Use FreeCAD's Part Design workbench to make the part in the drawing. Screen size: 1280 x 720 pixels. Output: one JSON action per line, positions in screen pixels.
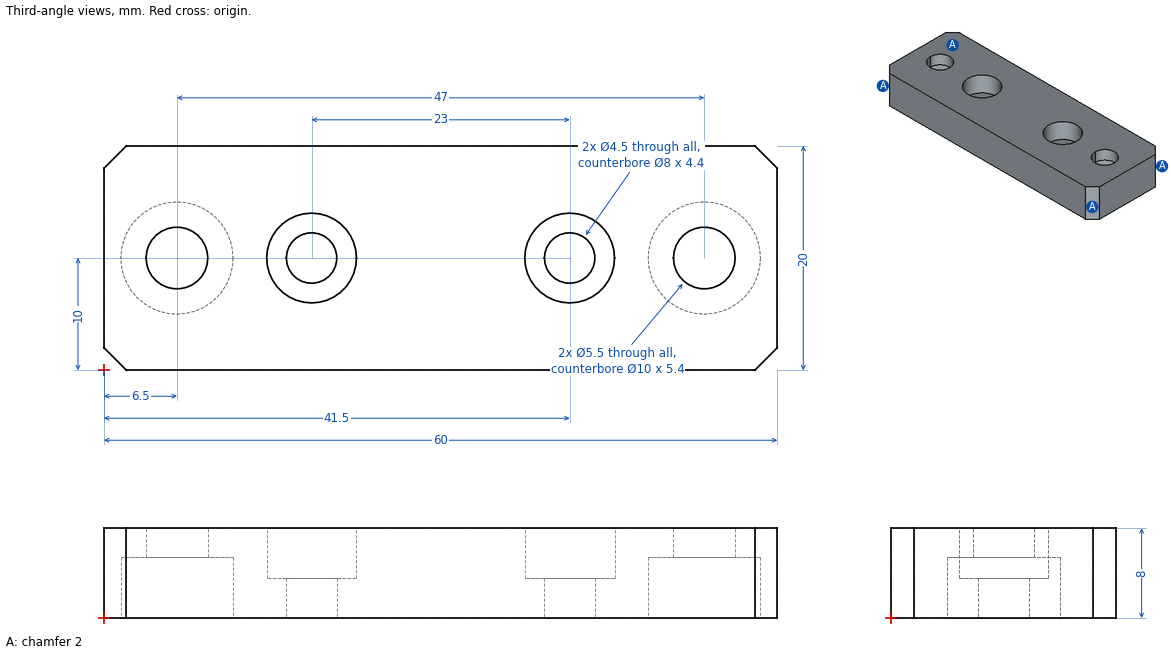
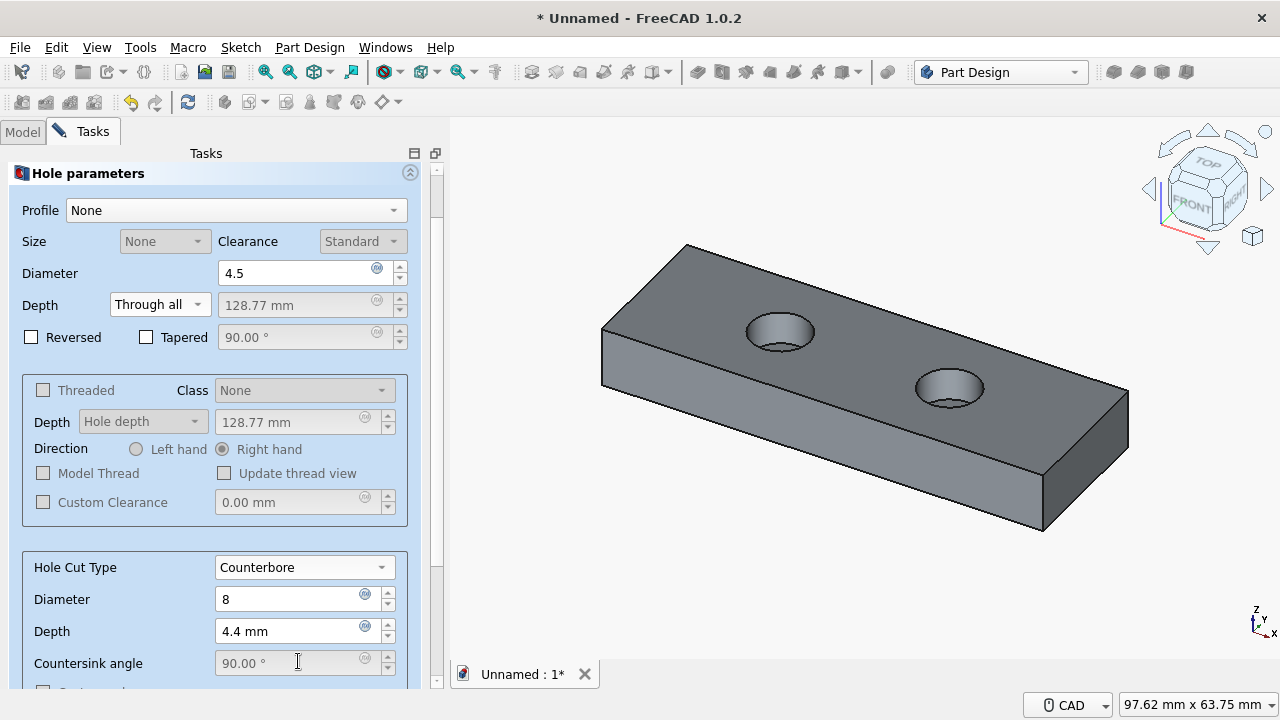
{"action": "scroll", "coordinate": [437, 426], "scroll_direction": "up", "scroll_amount": 2}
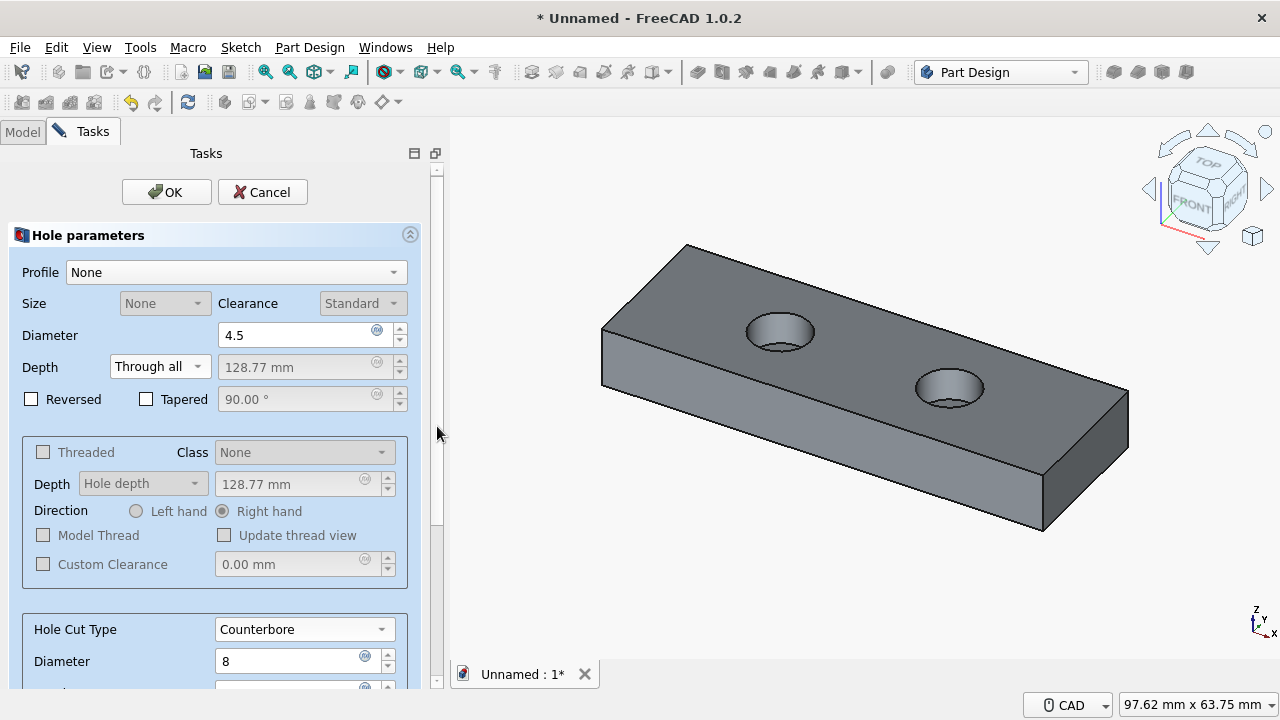
{"action": "left_click", "coordinate": [167, 192]}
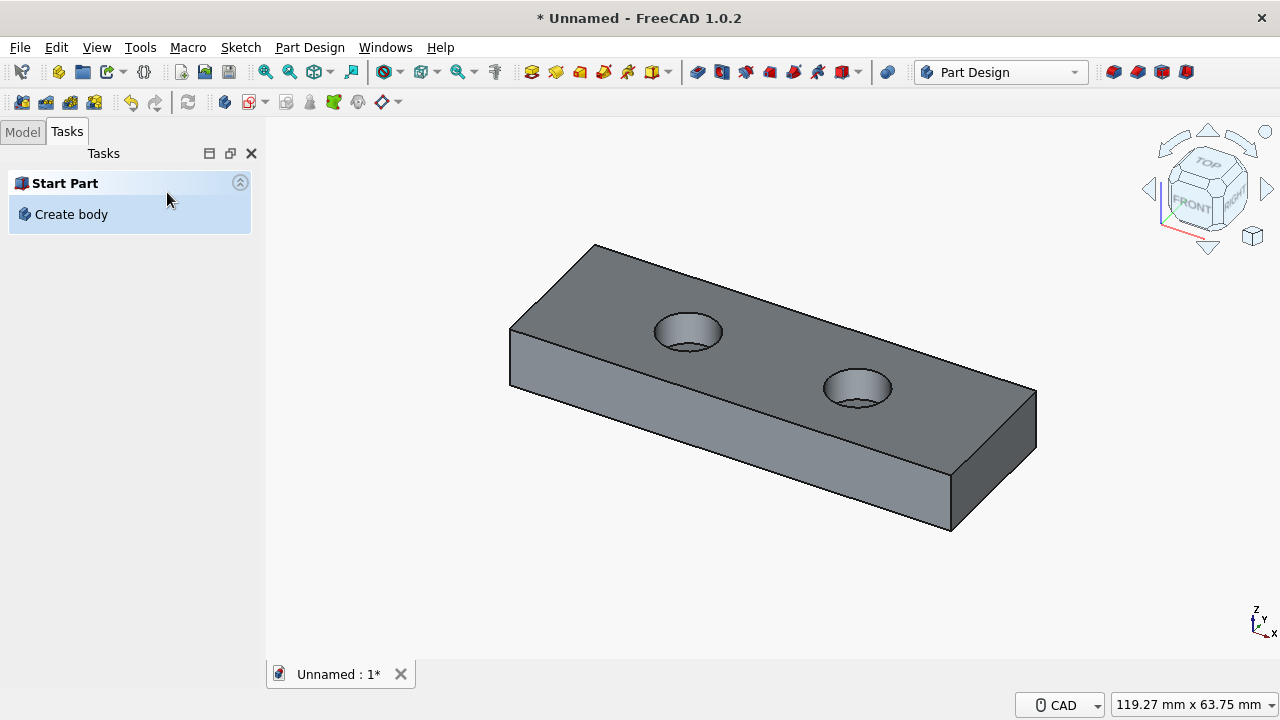
{"action": "left_click", "coordinate": [250, 102]}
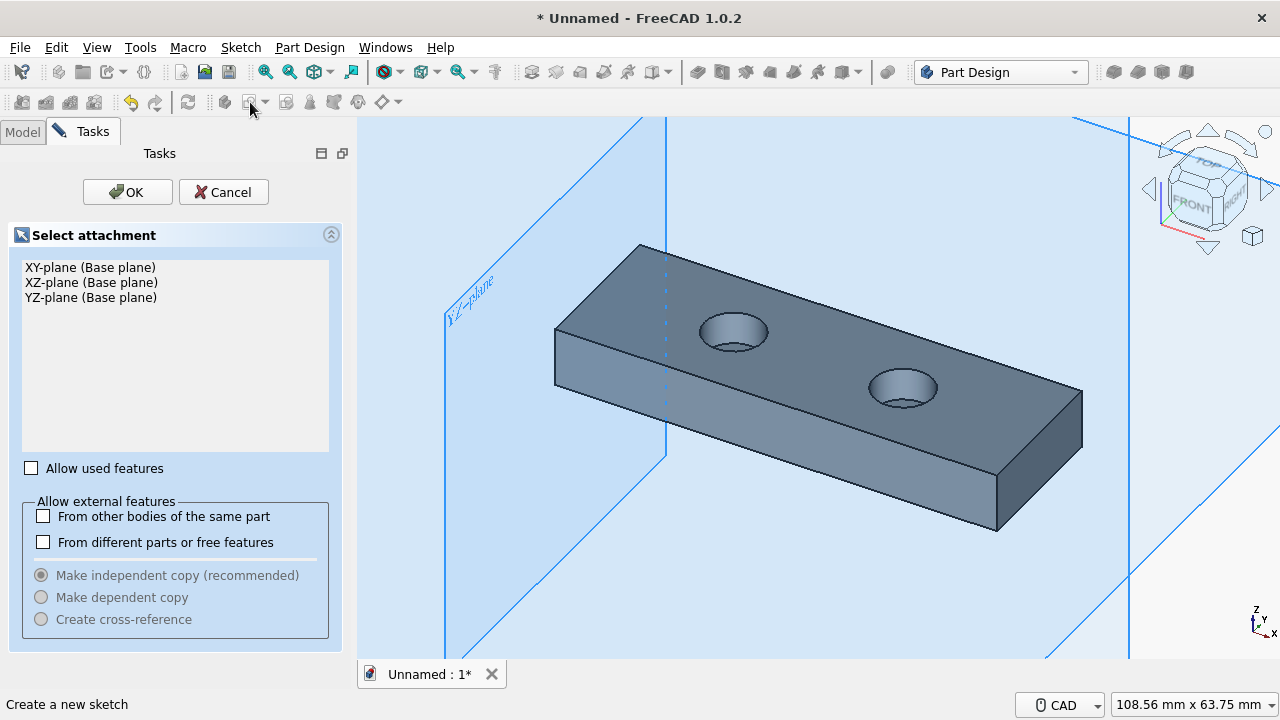
{"action": "left_click", "coordinate": [82, 268]}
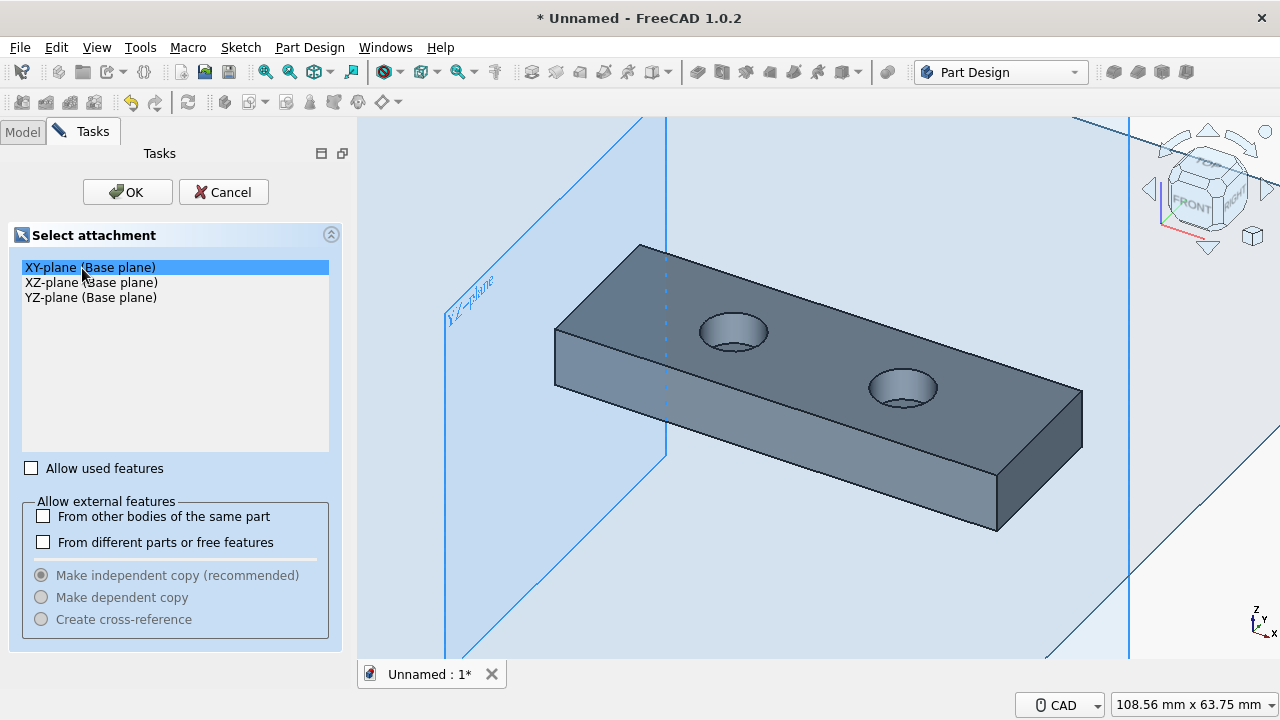
{"action": "left_click", "coordinate": [128, 192]}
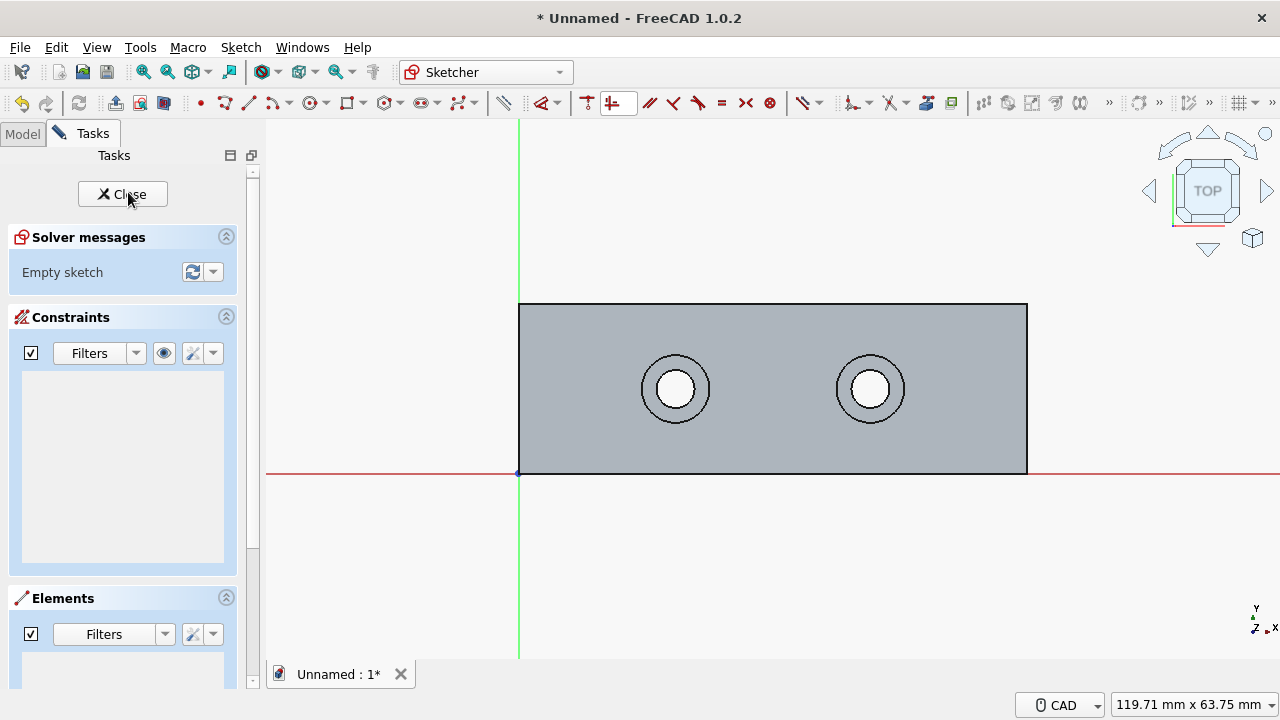
{"action": "left_click", "coordinate": [164, 104]}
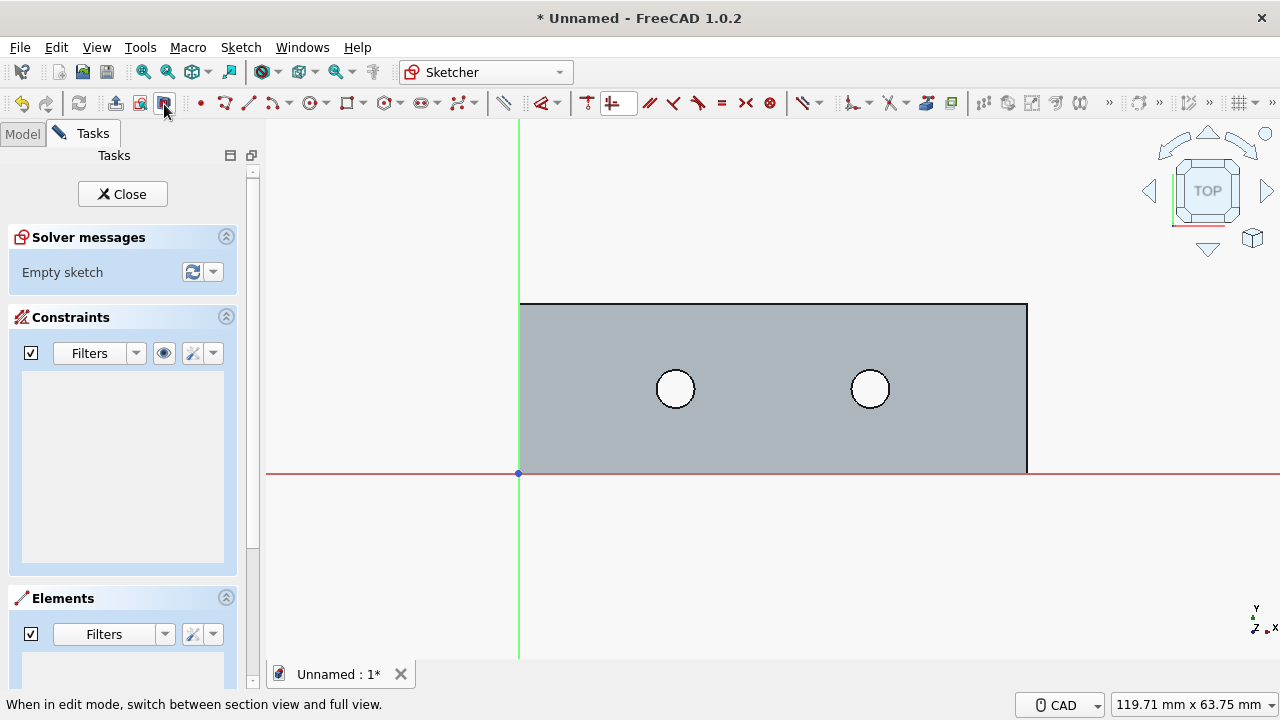
{"action": "key", "text": "g c"}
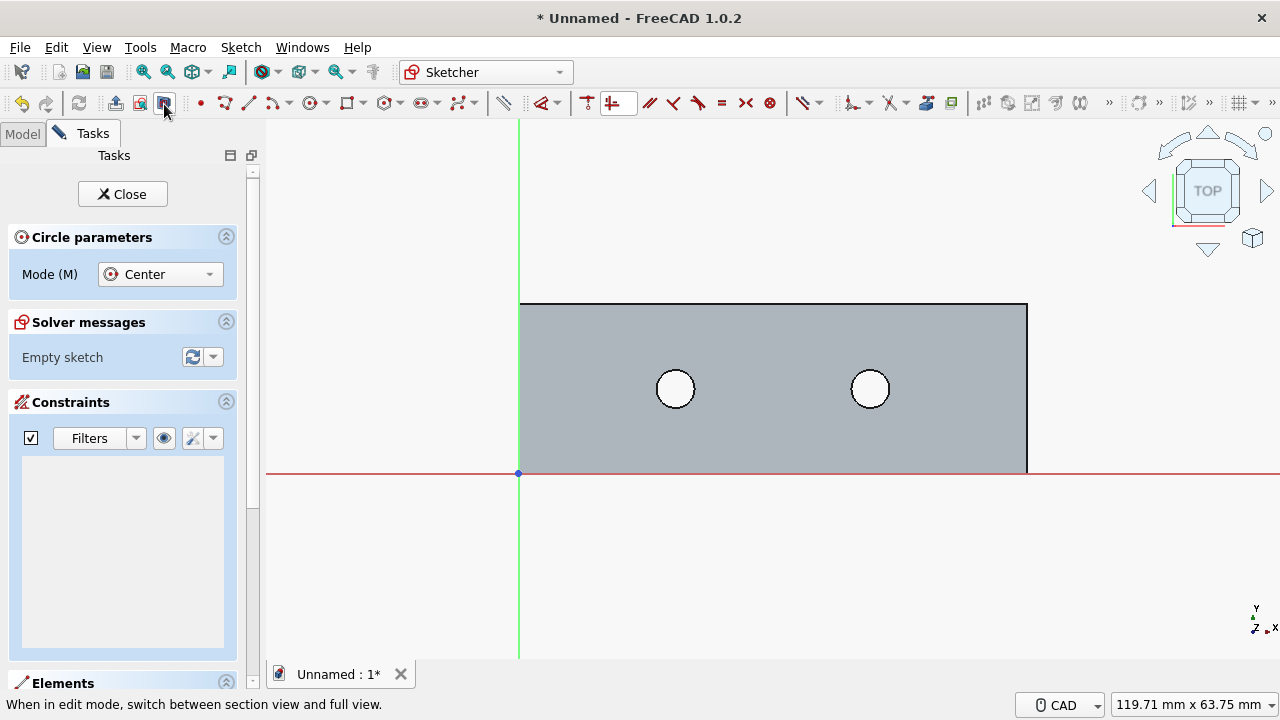
{"action": "left_click", "coordinate": [972, 389]}
{"action": "mouse_move", "coordinate": [989, 373]}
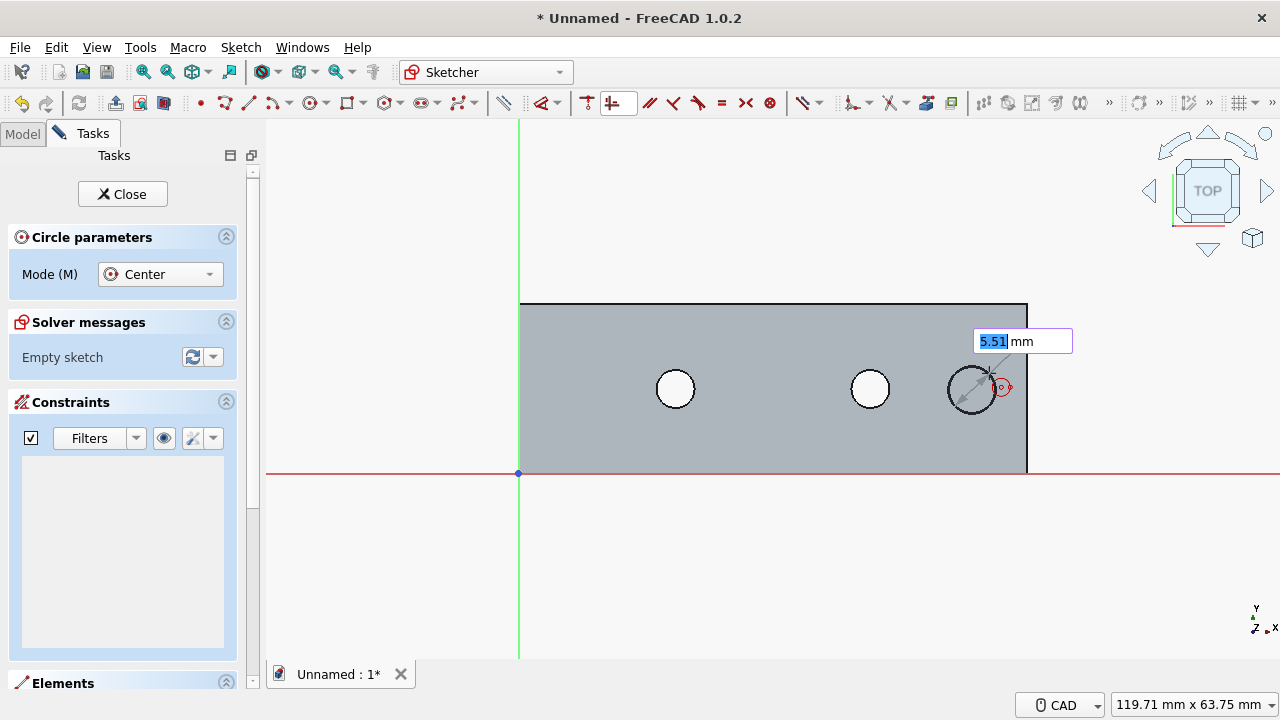
{"action": "type", "text": "5.5"}
{"action": "key", "text": "Return"}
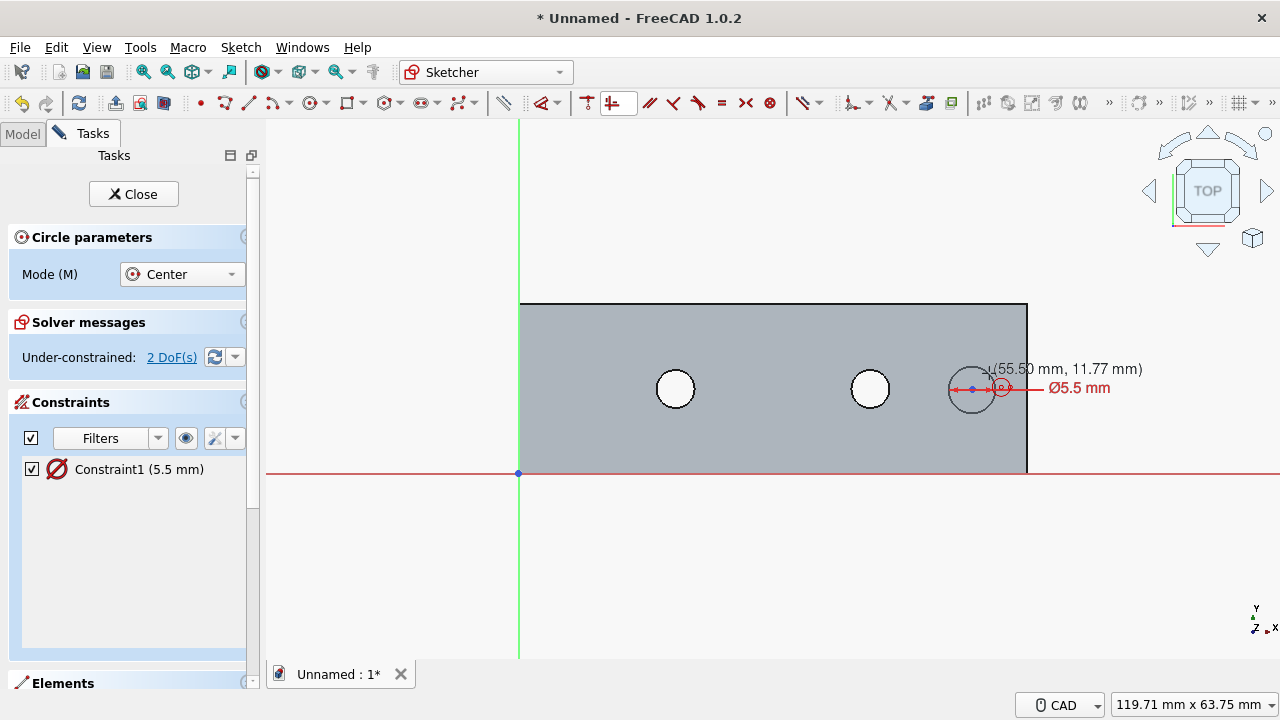
{"action": "left_click", "coordinate": [574, 389]}
{"action": "mouse_move", "coordinate": [590, 373]}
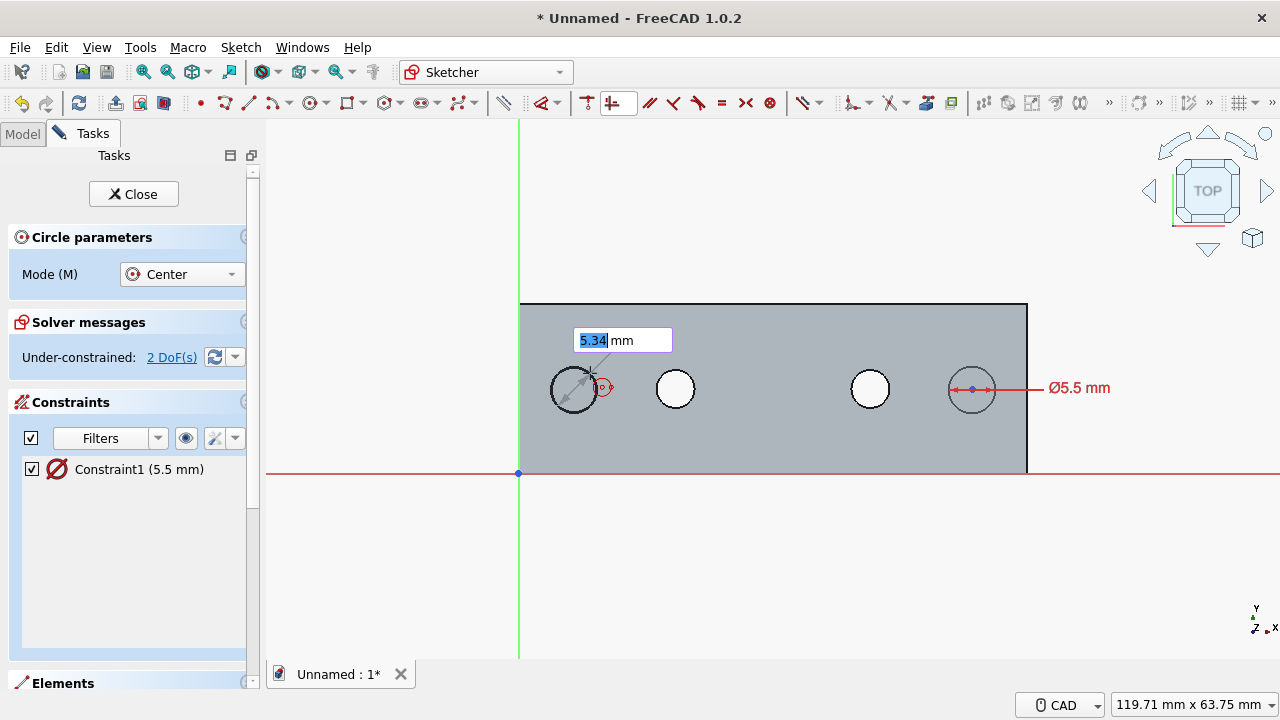
{"action": "type", "text": "5.5"}
{"action": "key", "text": "Return"}
{"action": "key", "text": "Escape"}